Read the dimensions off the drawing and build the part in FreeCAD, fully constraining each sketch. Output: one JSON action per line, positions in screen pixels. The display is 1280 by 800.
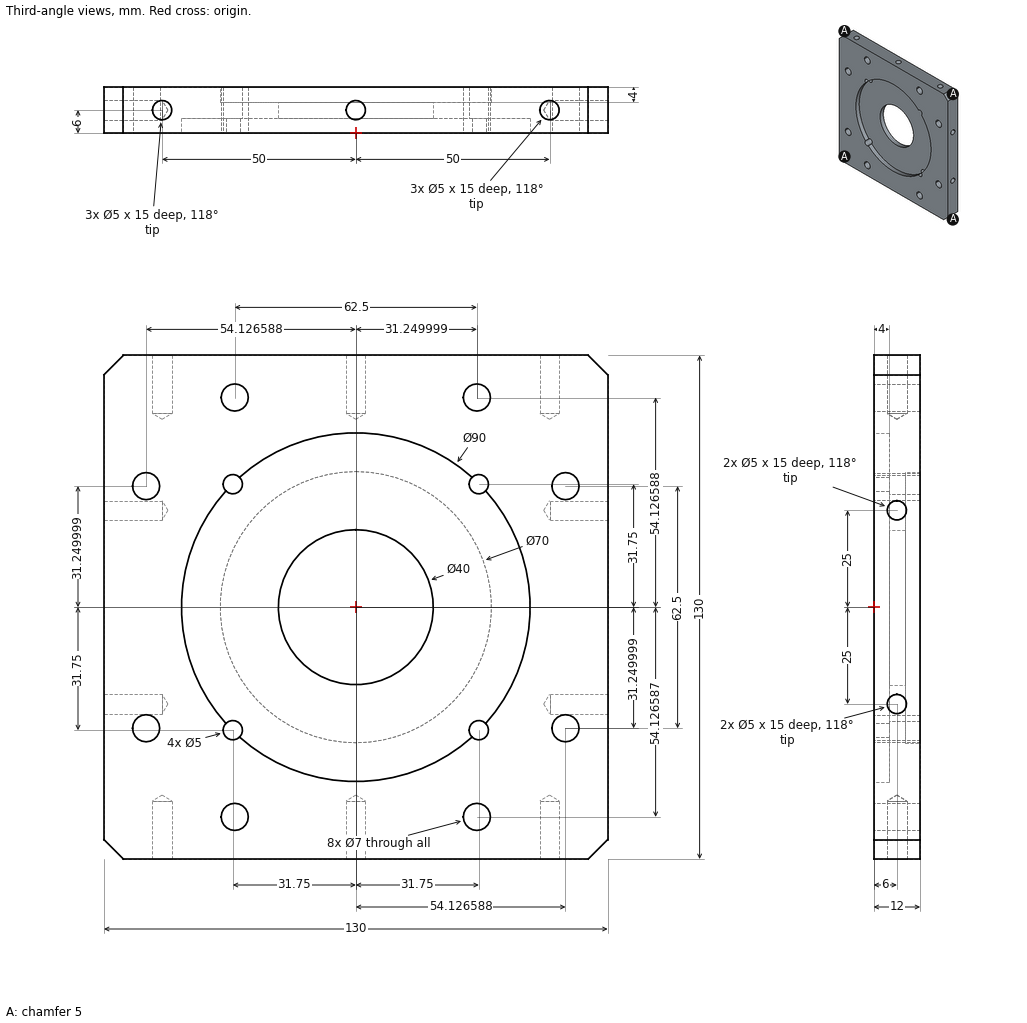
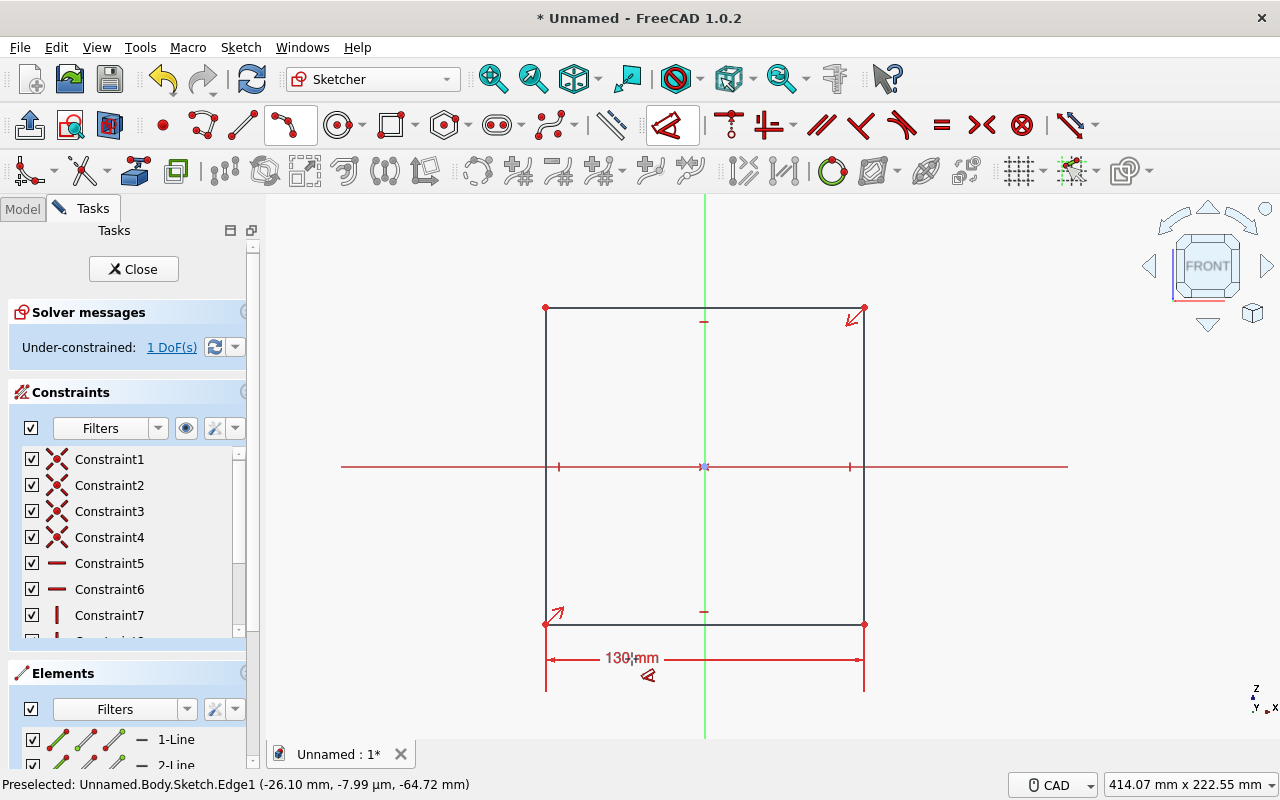
{"action": "left_click", "coordinate": [864, 530]}
{"action": "left_click", "coordinate": [898, 394]}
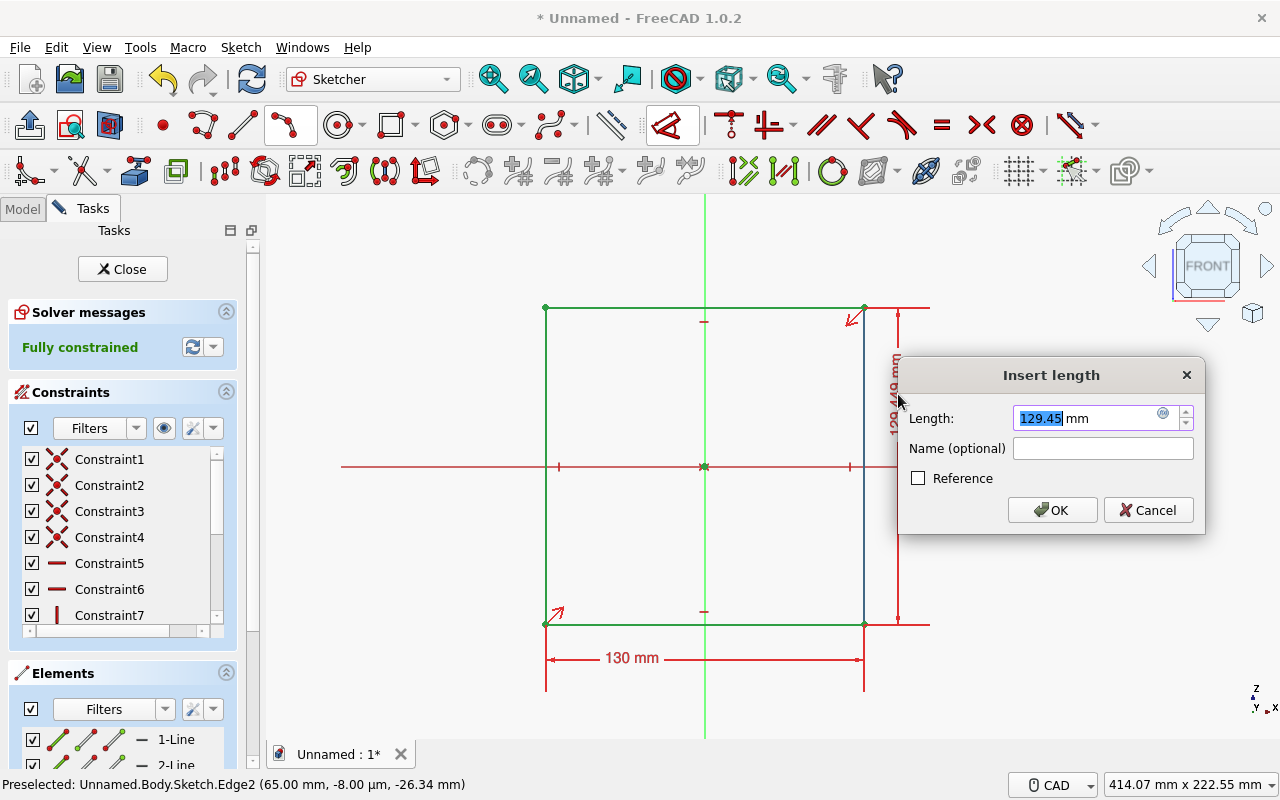
{"action": "type", "text": "130"}
{"action": "key", "text": "Return"}
{"action": "key", "text": "Escape"}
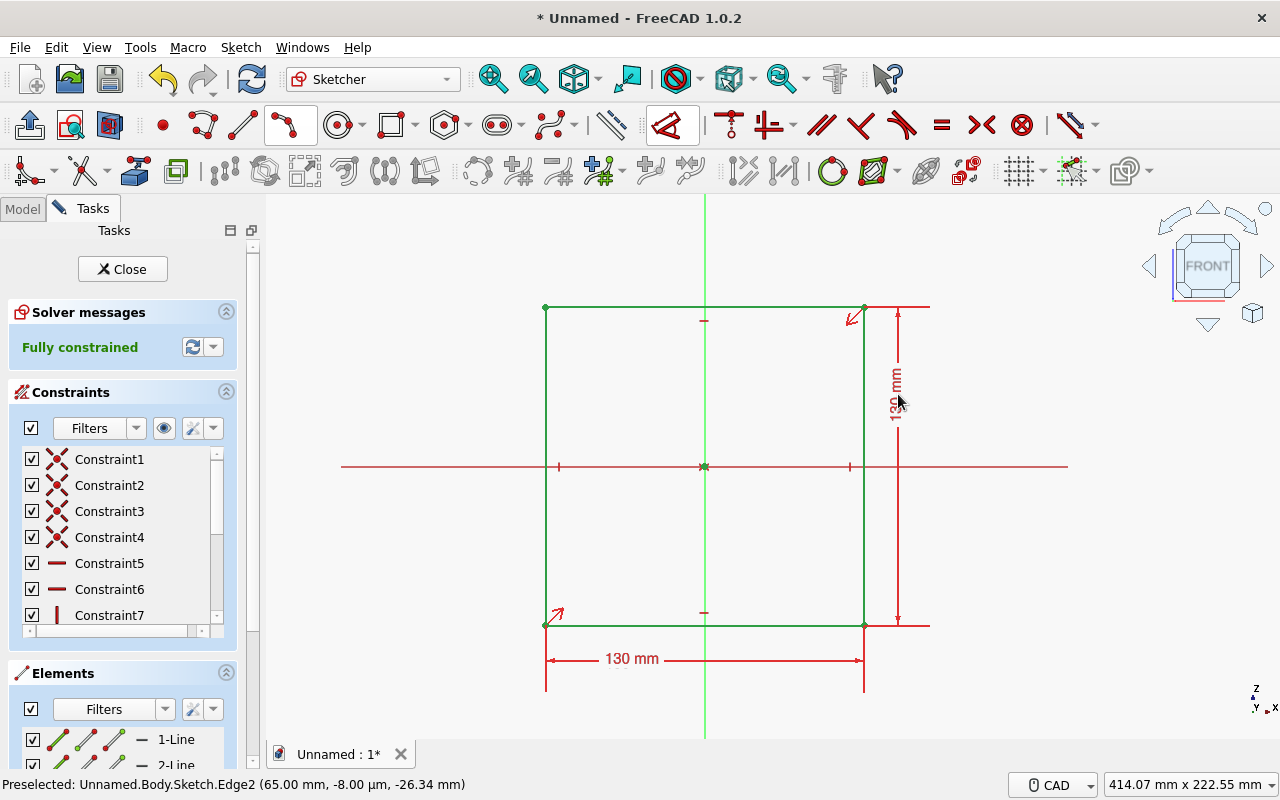
{"action": "left_click", "coordinate": [123, 269]}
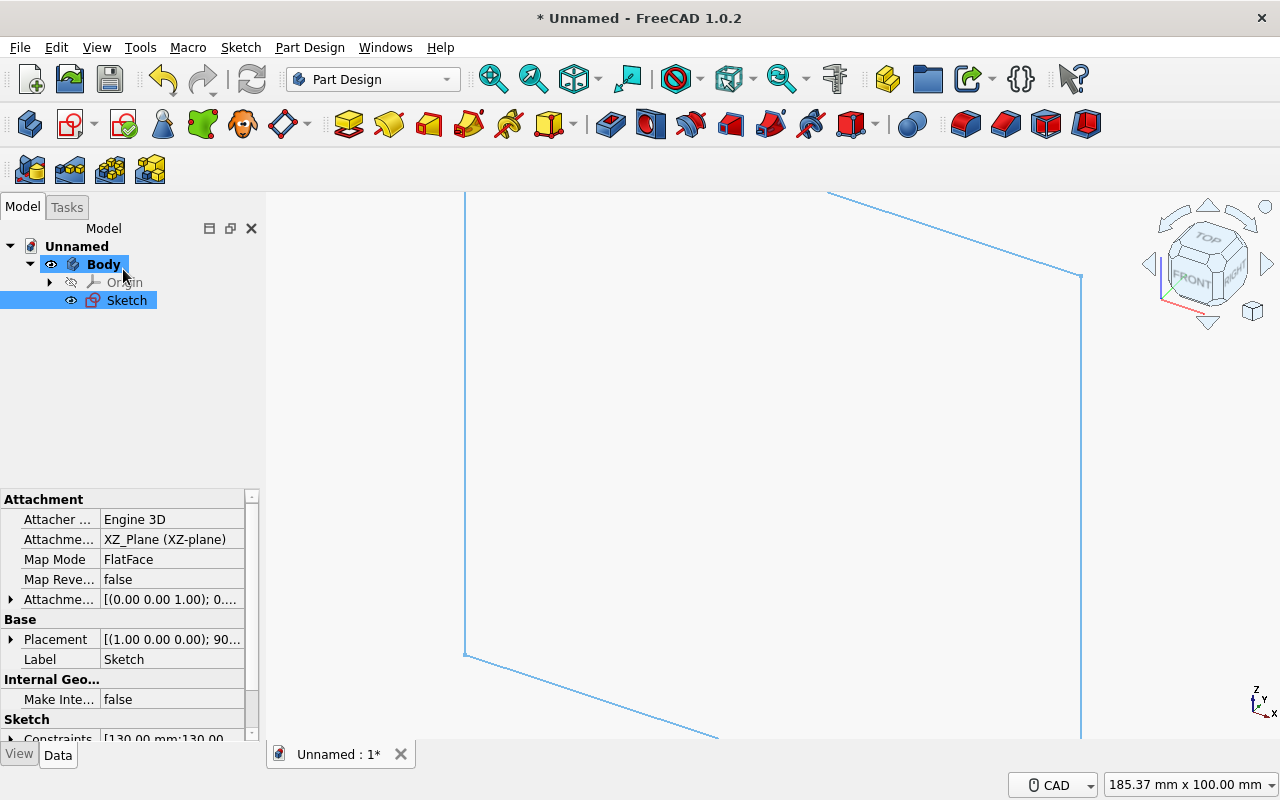
{"action": "left_click", "coordinate": [350, 124]}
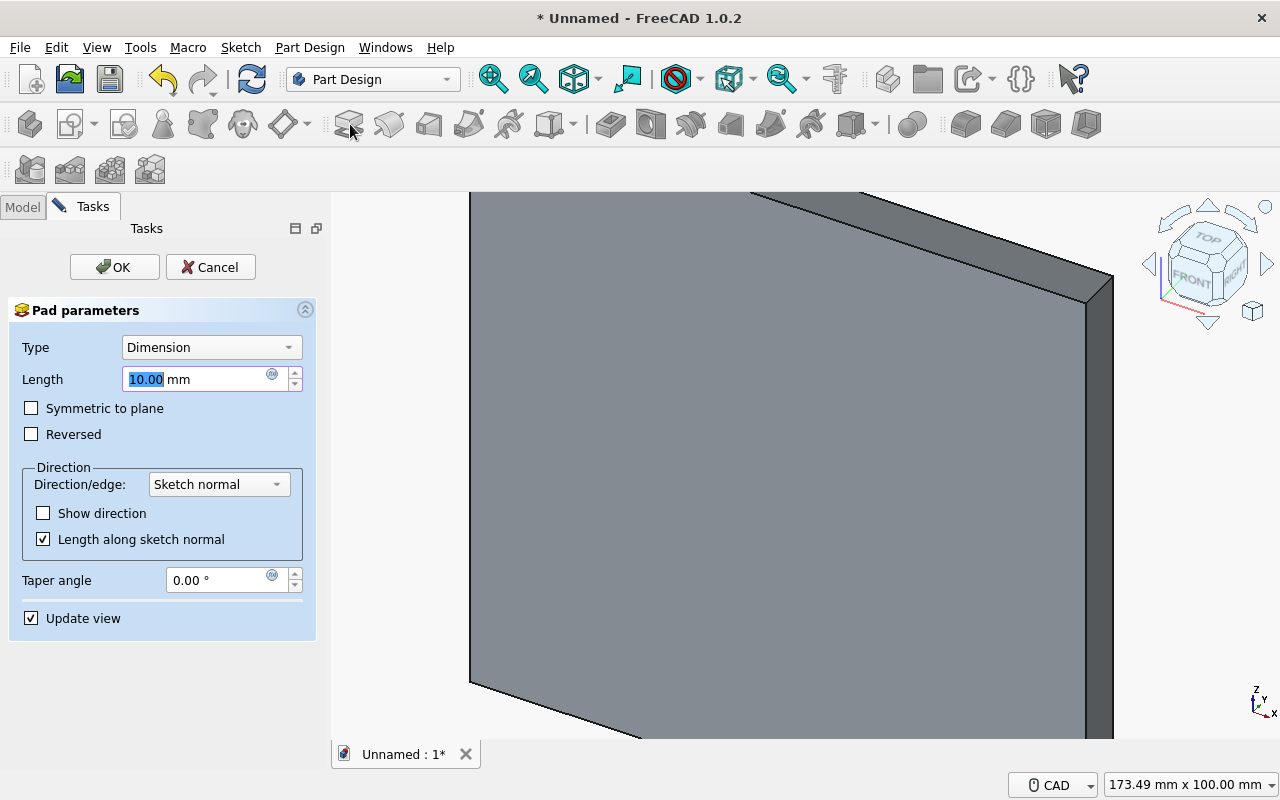
{"action": "type", "text": "12"}
{"action": "key", "text": "Tab"}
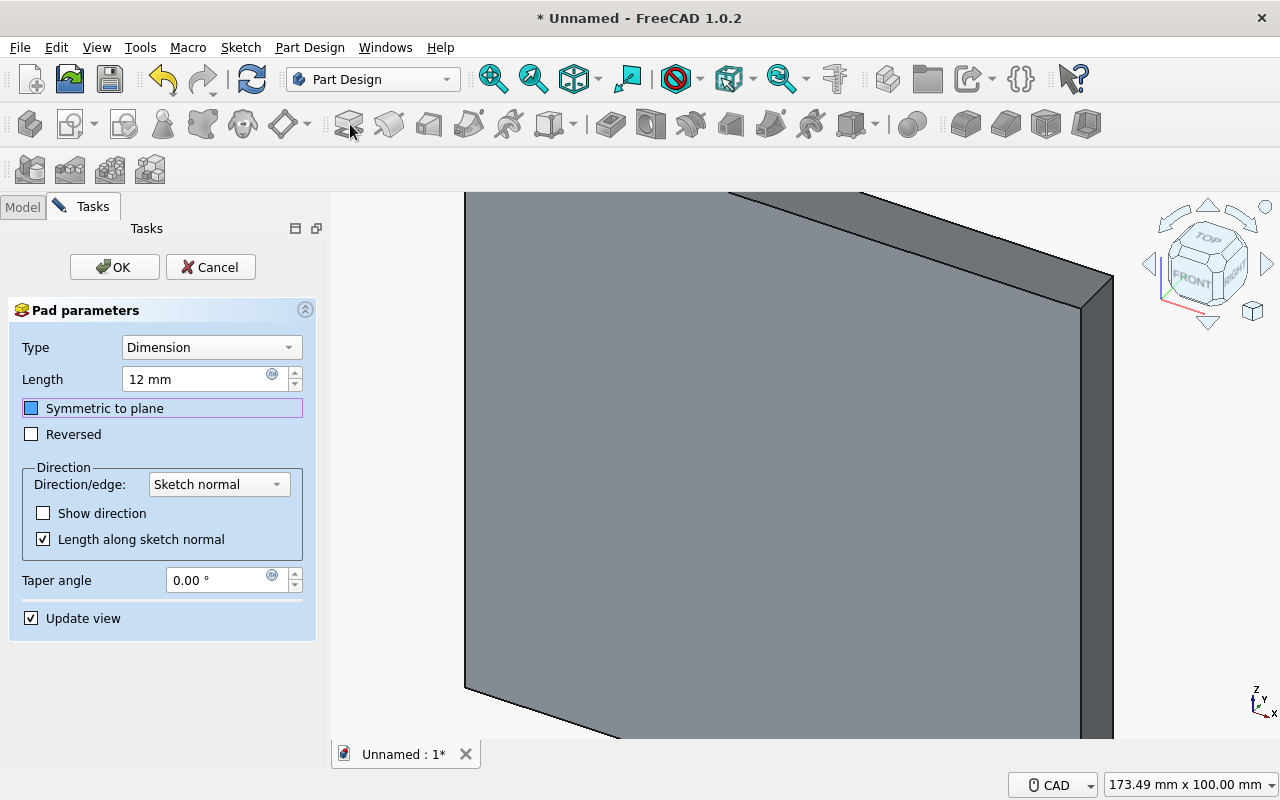
{"action": "left_click", "coordinate": [30, 434]}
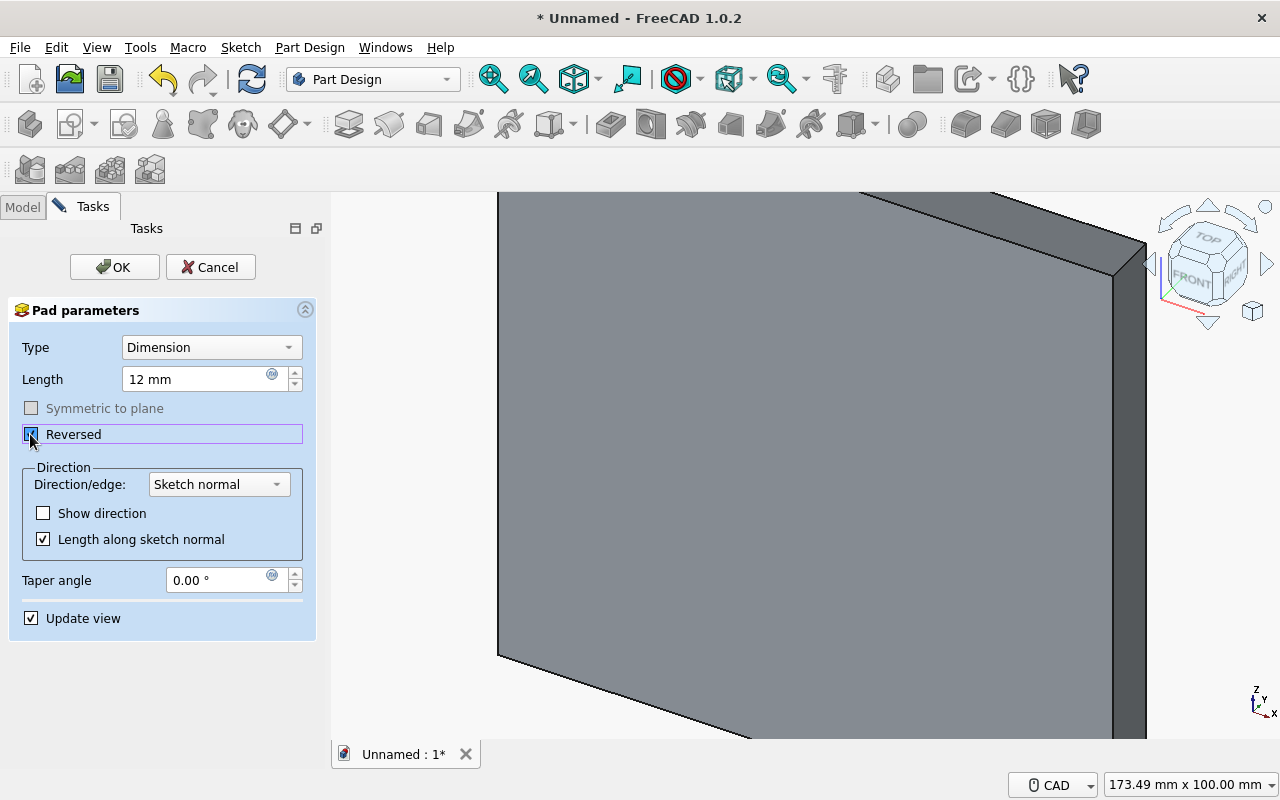
{"action": "left_click", "coordinate": [115, 267]}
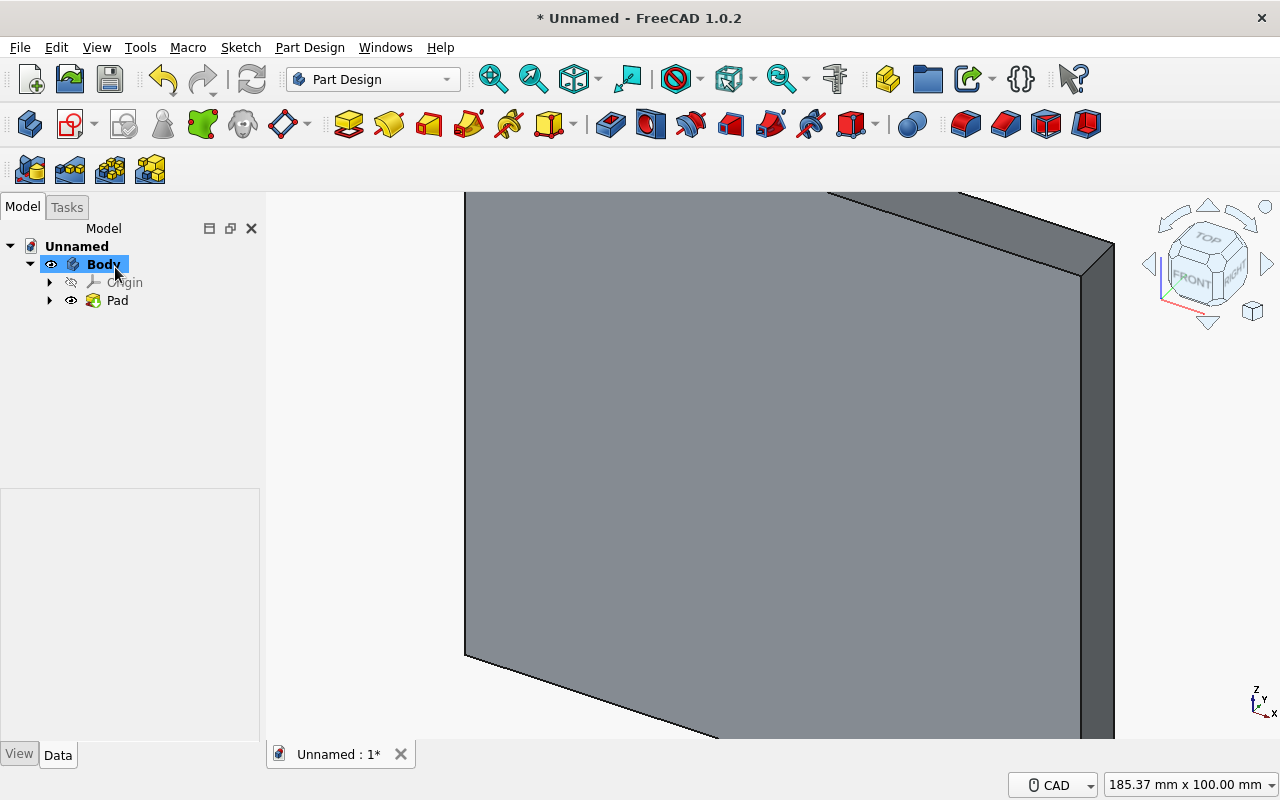
{"action": "key", "text": "v f"}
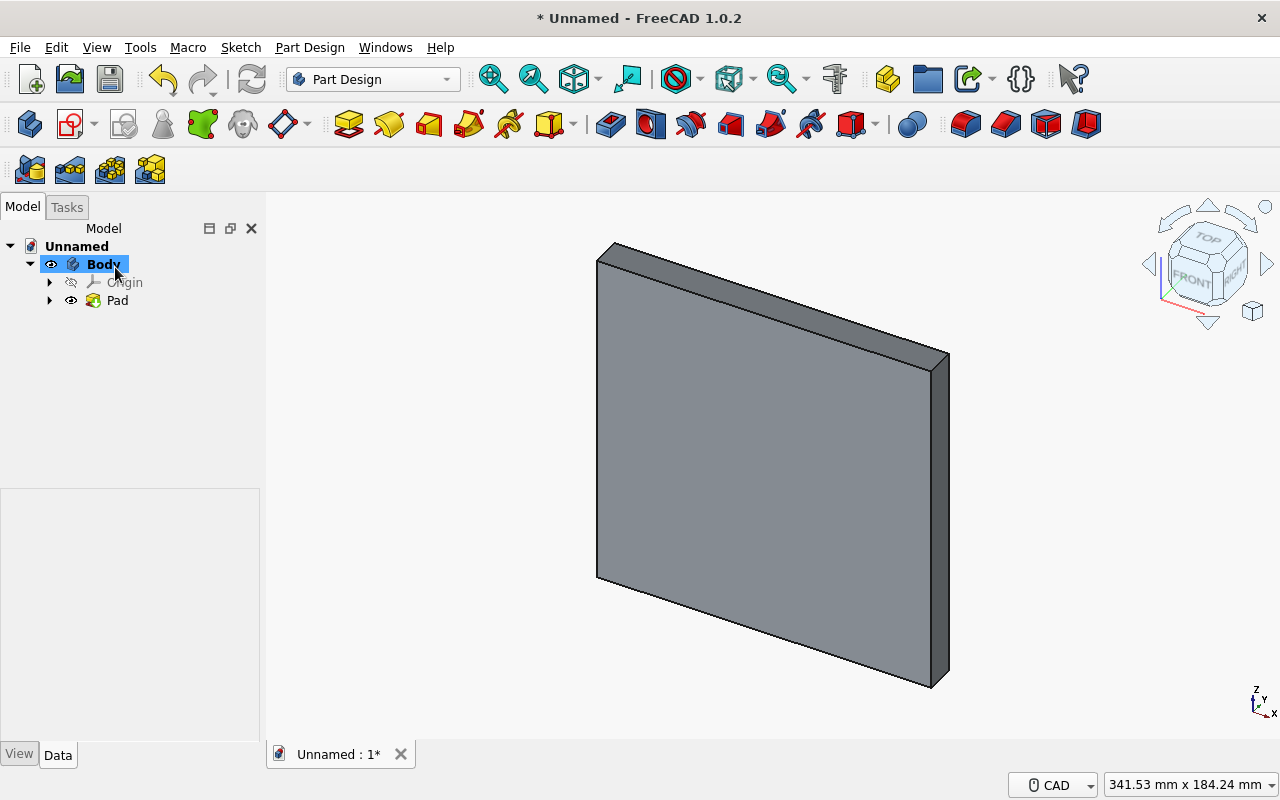
{"action": "key", "text": "4"}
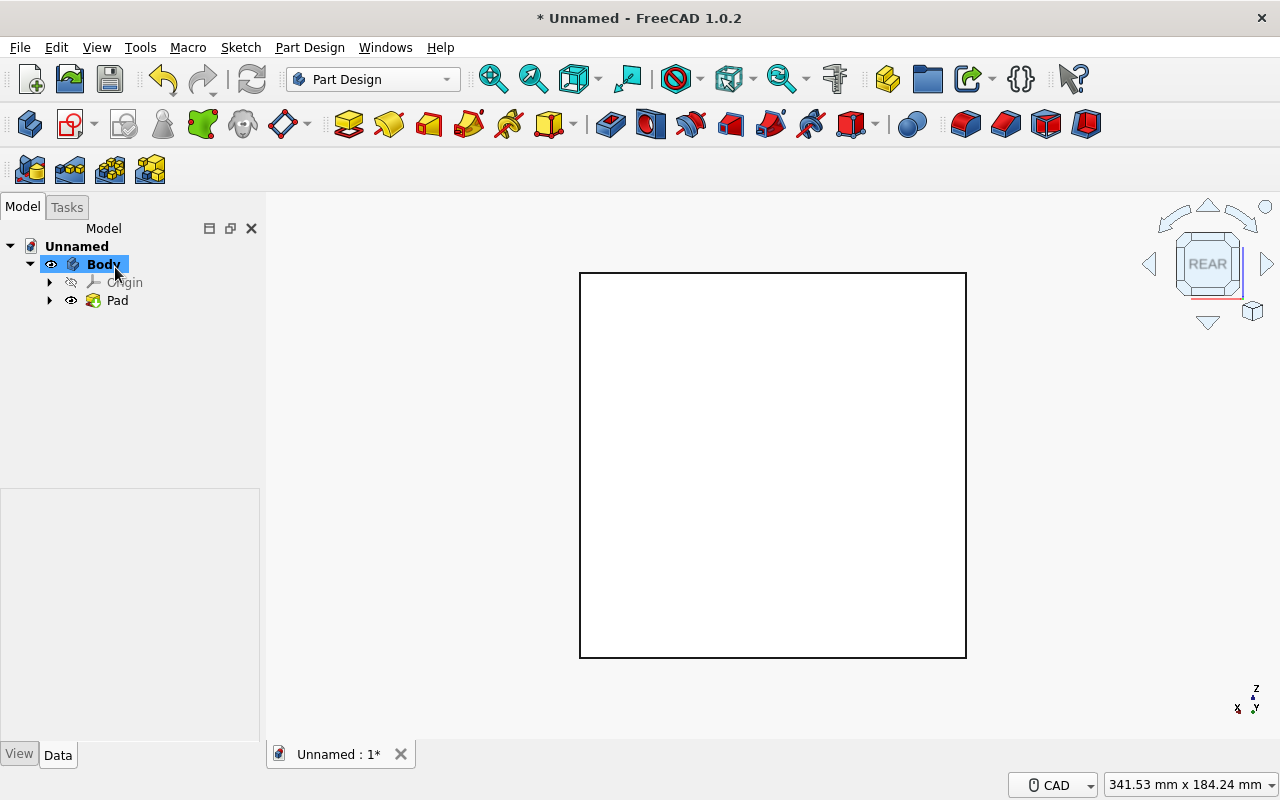
{"action": "left_click", "coordinate": [773, 465]}